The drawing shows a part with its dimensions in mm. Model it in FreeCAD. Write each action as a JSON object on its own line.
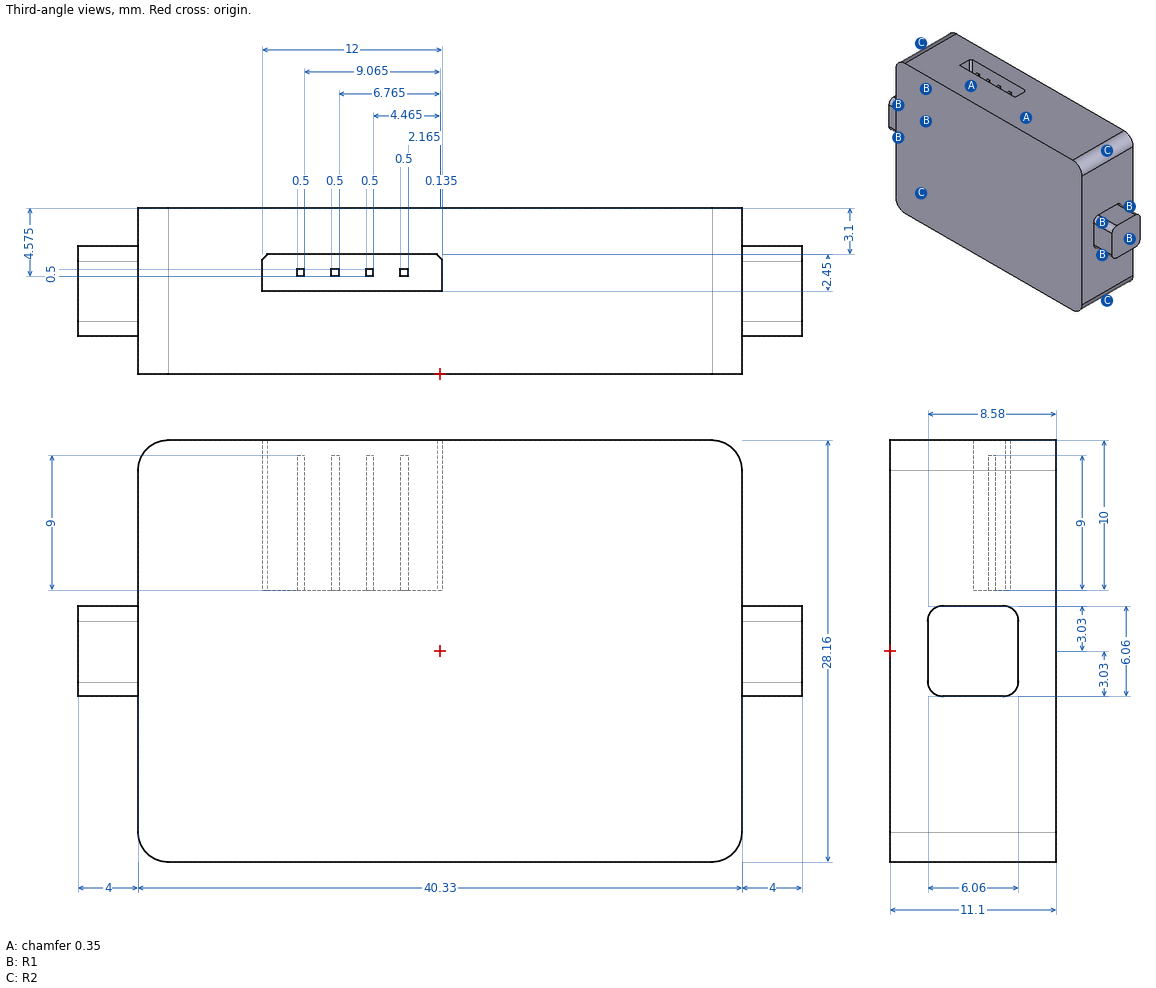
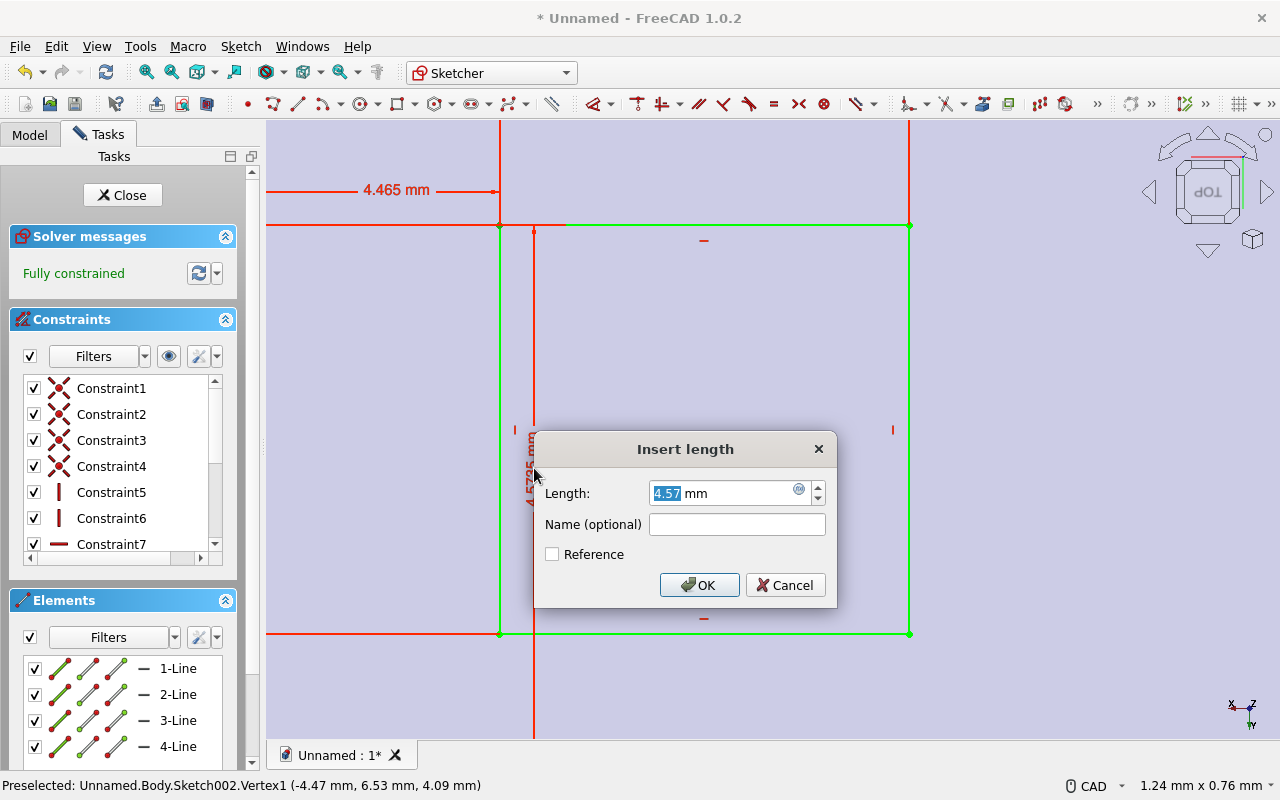
{"action": "type", "text": "4.575"}
{"action": "key", "text": "Return"}
{"action": "key", "text": "Escape"}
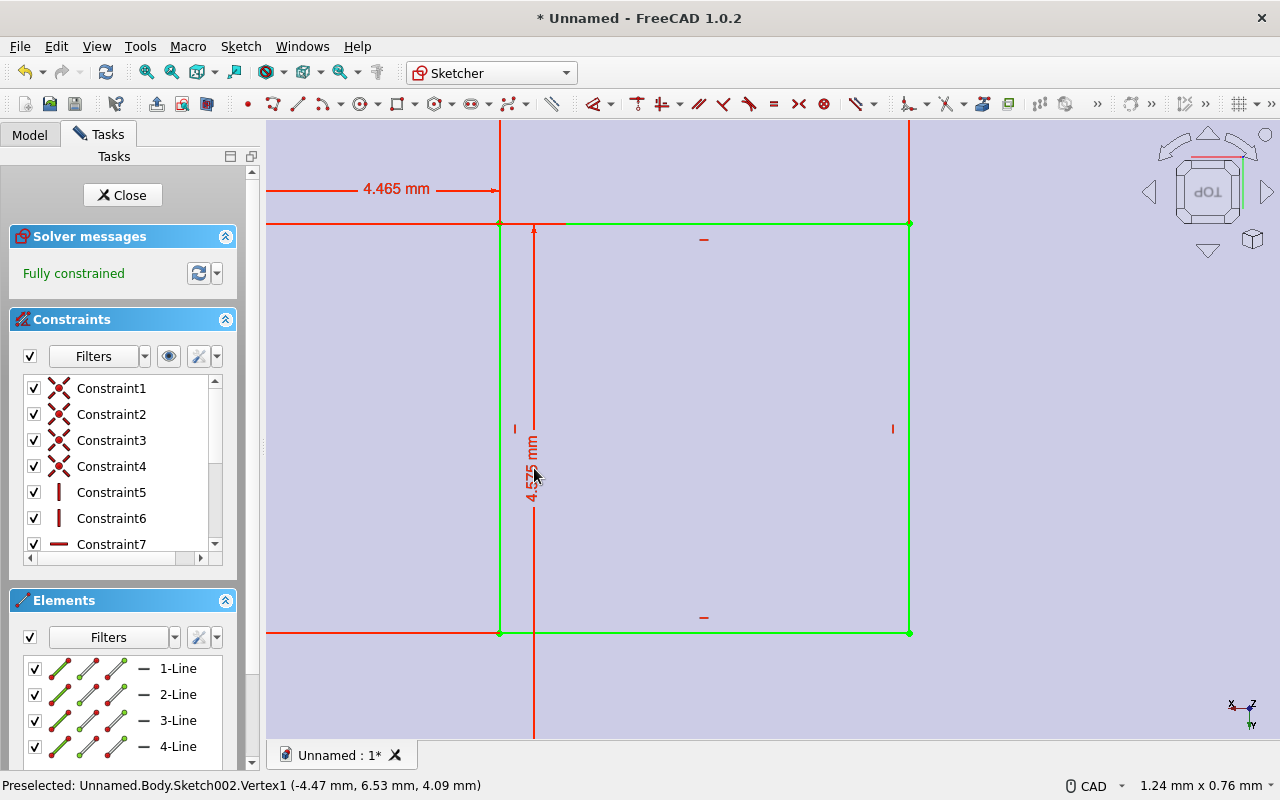
{"action": "left_click", "coordinate": [123, 195]}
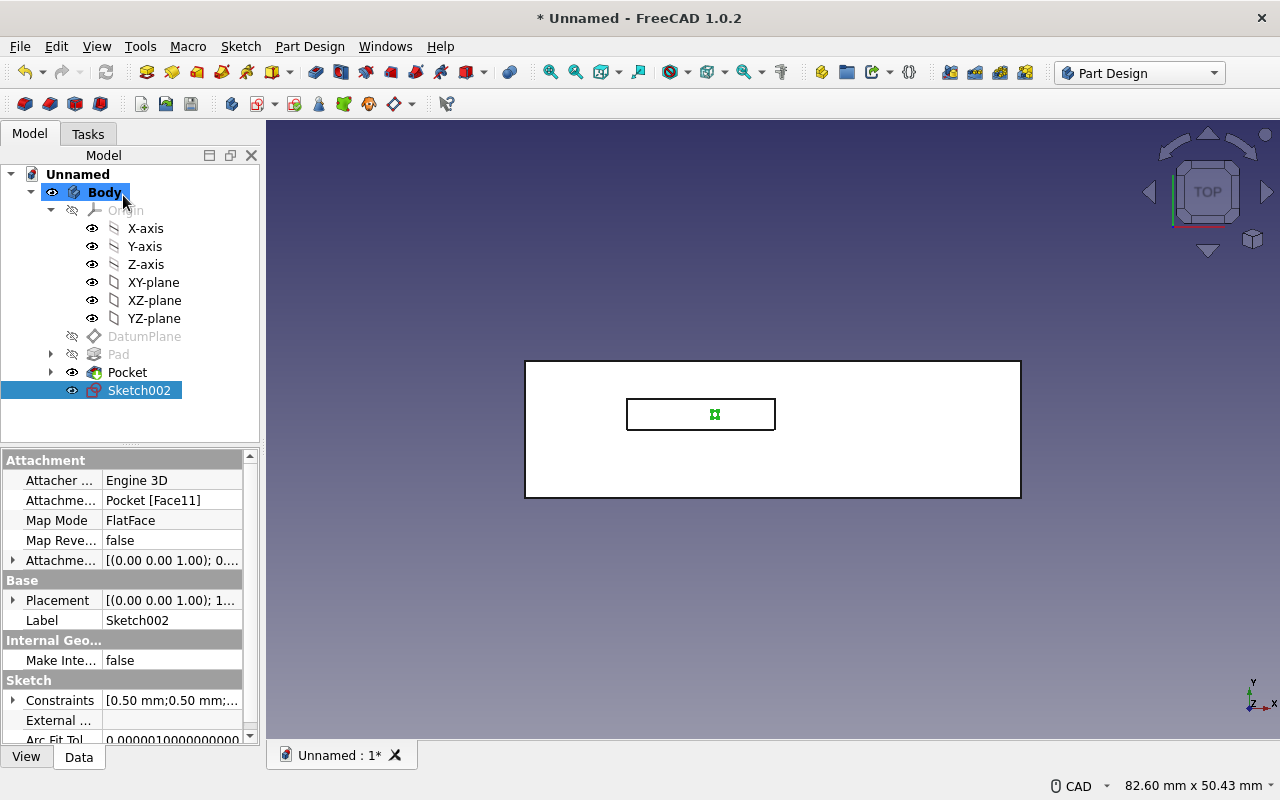
{"action": "left_click", "coordinate": [147, 72]}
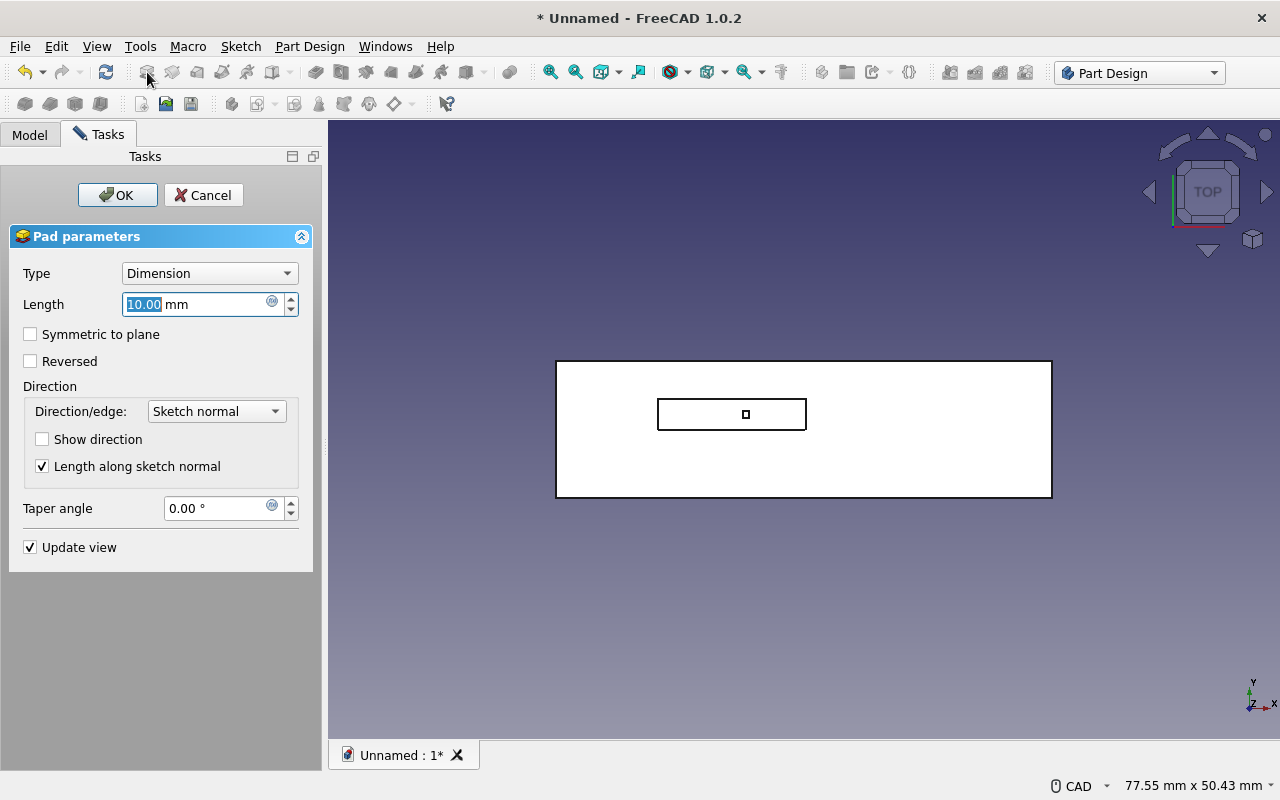
{"action": "type", "text": "9"}
{"action": "key", "text": "Tab"}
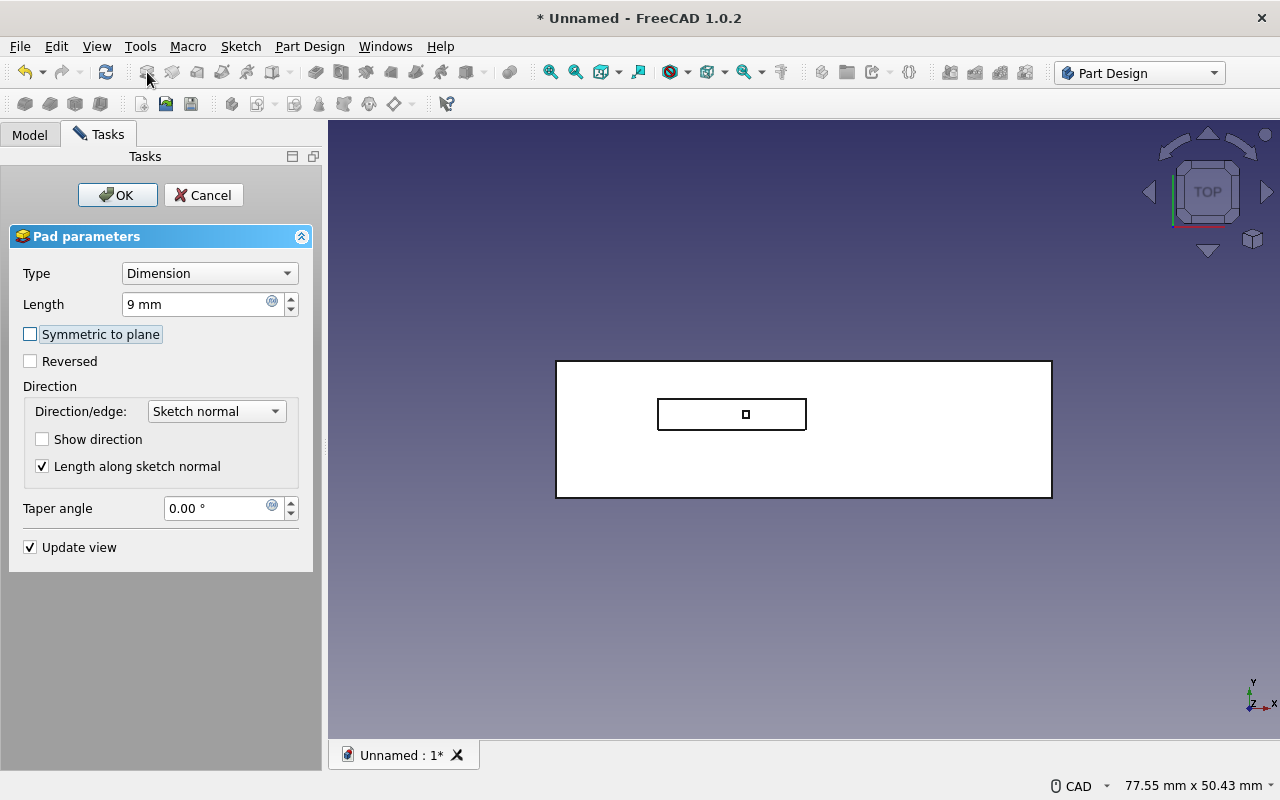
{"action": "left_click", "coordinate": [118, 195]}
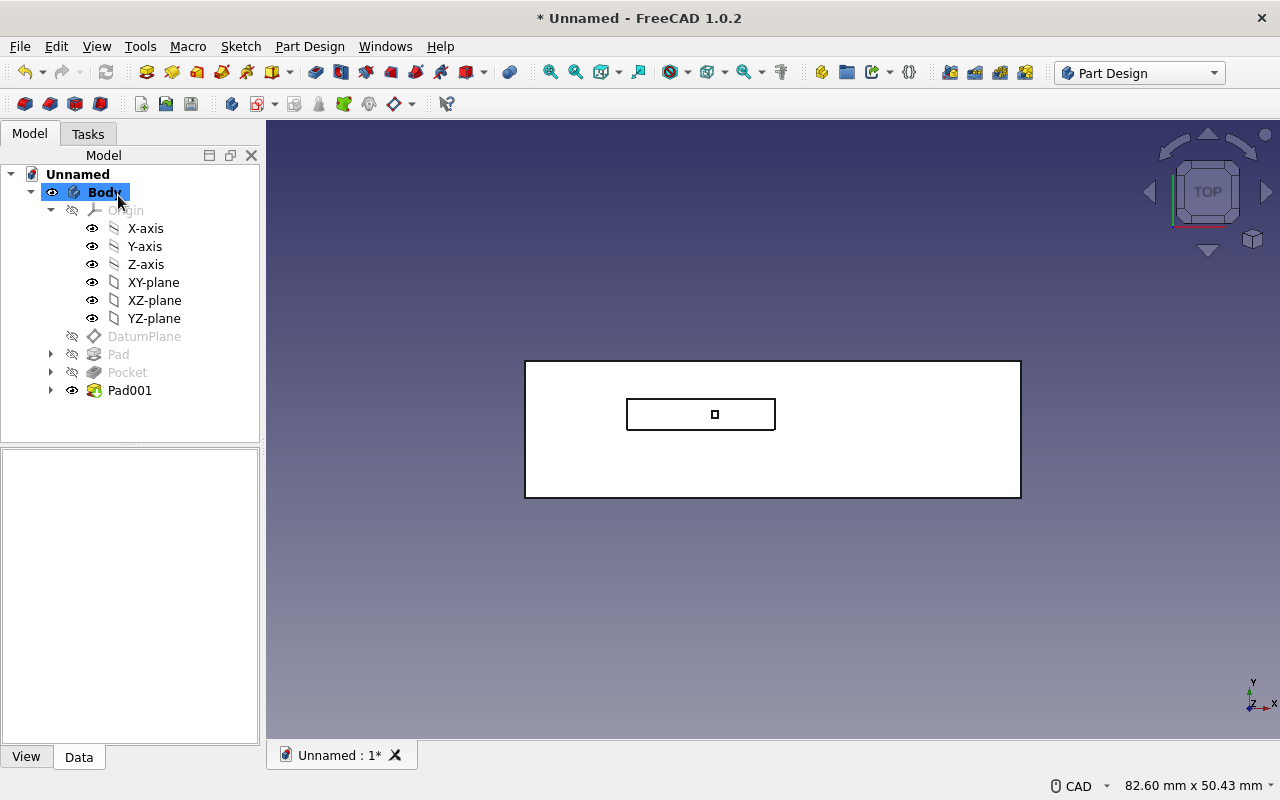
{"action": "left_click", "coordinate": [743, 413]}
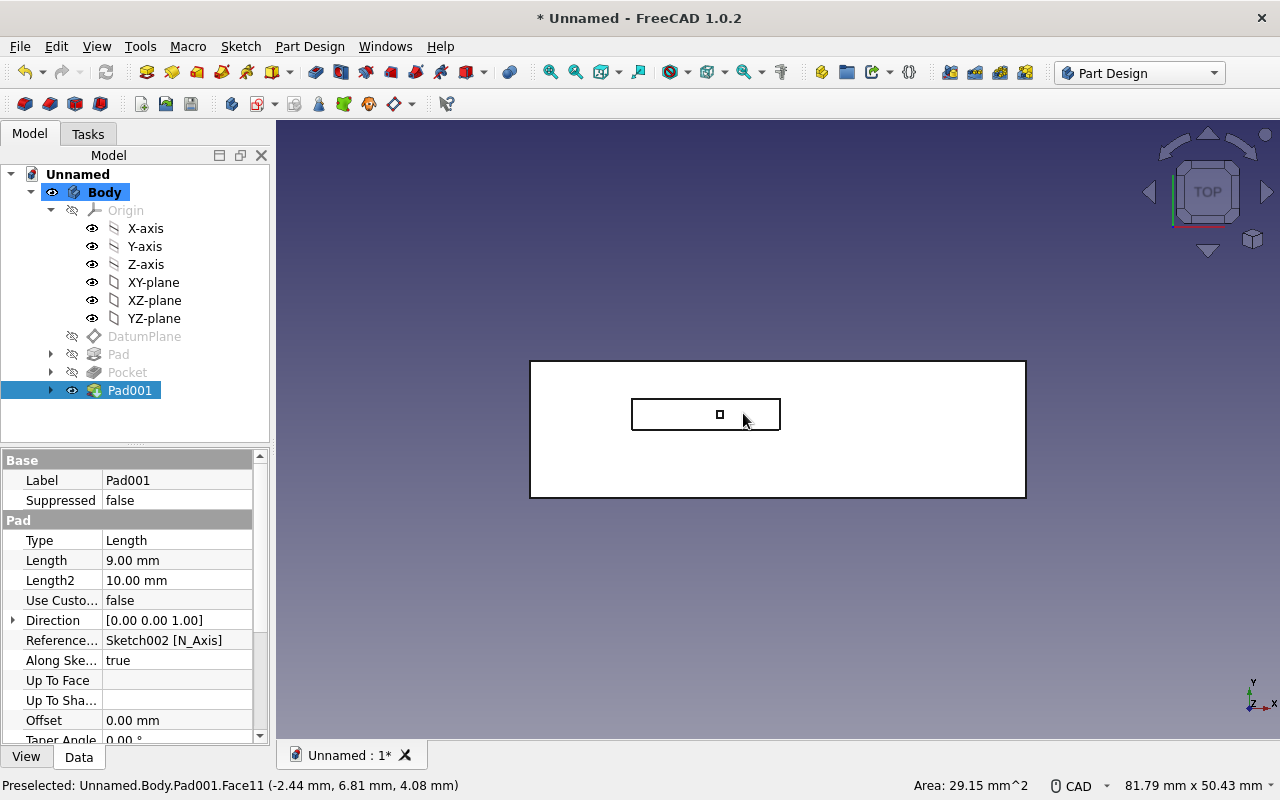
{"action": "left_click", "coordinate": [256, 104]}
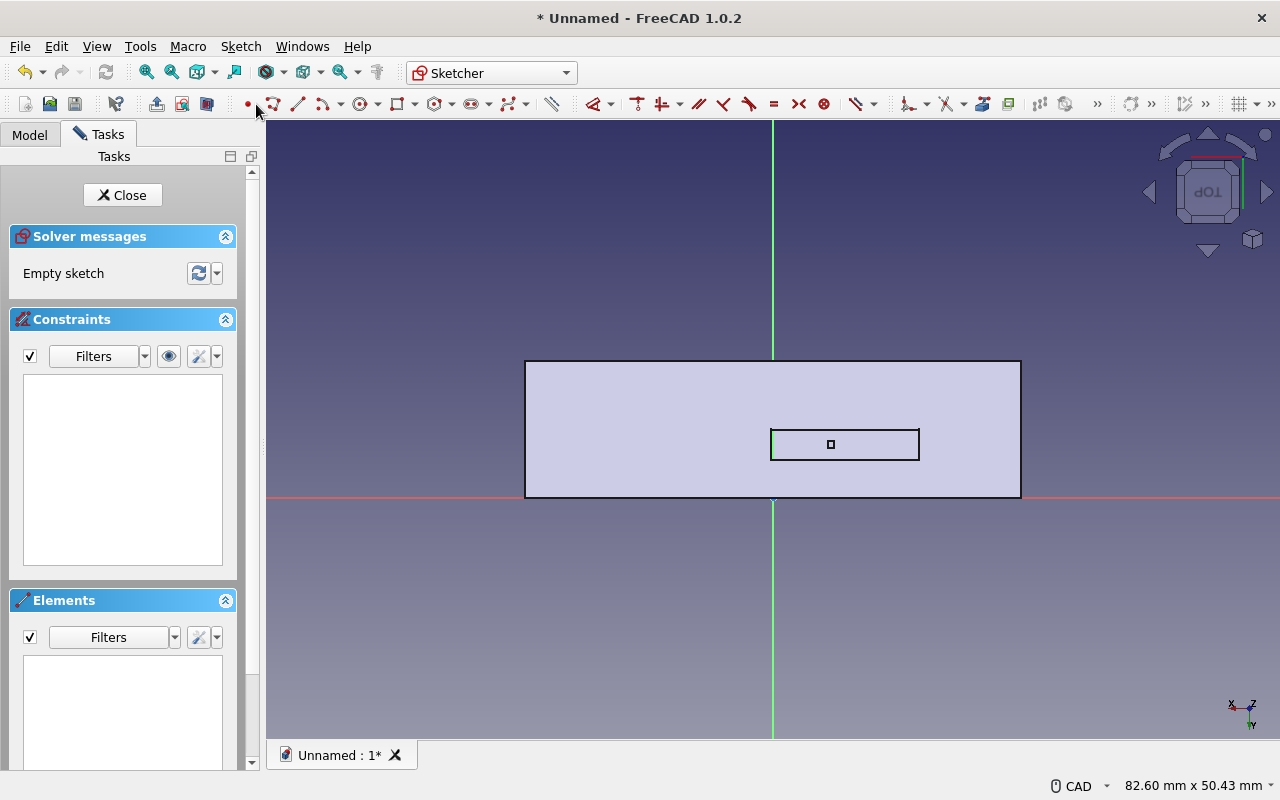
{"action": "left_click", "coordinate": [207, 104]}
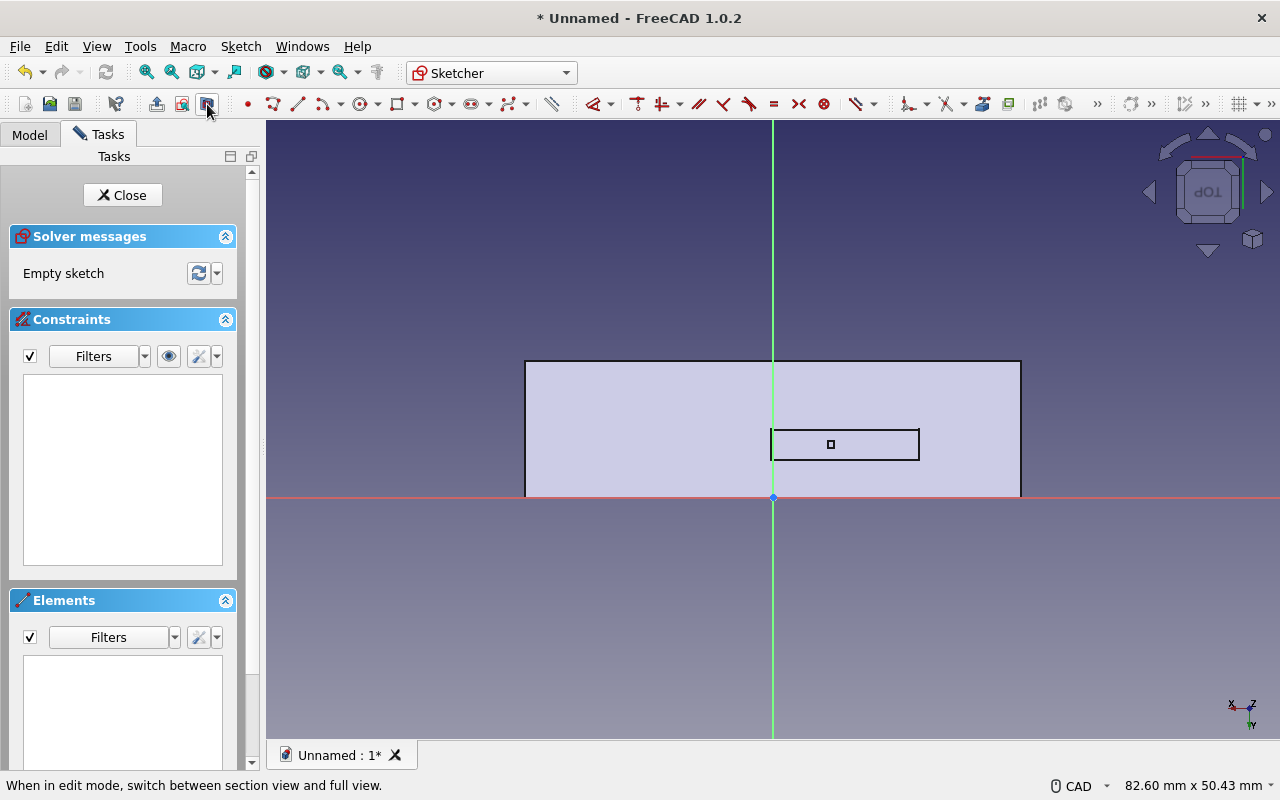
{"action": "scroll", "coordinate": [897, 445], "scroll_direction": "up", "scroll_amount": 15}